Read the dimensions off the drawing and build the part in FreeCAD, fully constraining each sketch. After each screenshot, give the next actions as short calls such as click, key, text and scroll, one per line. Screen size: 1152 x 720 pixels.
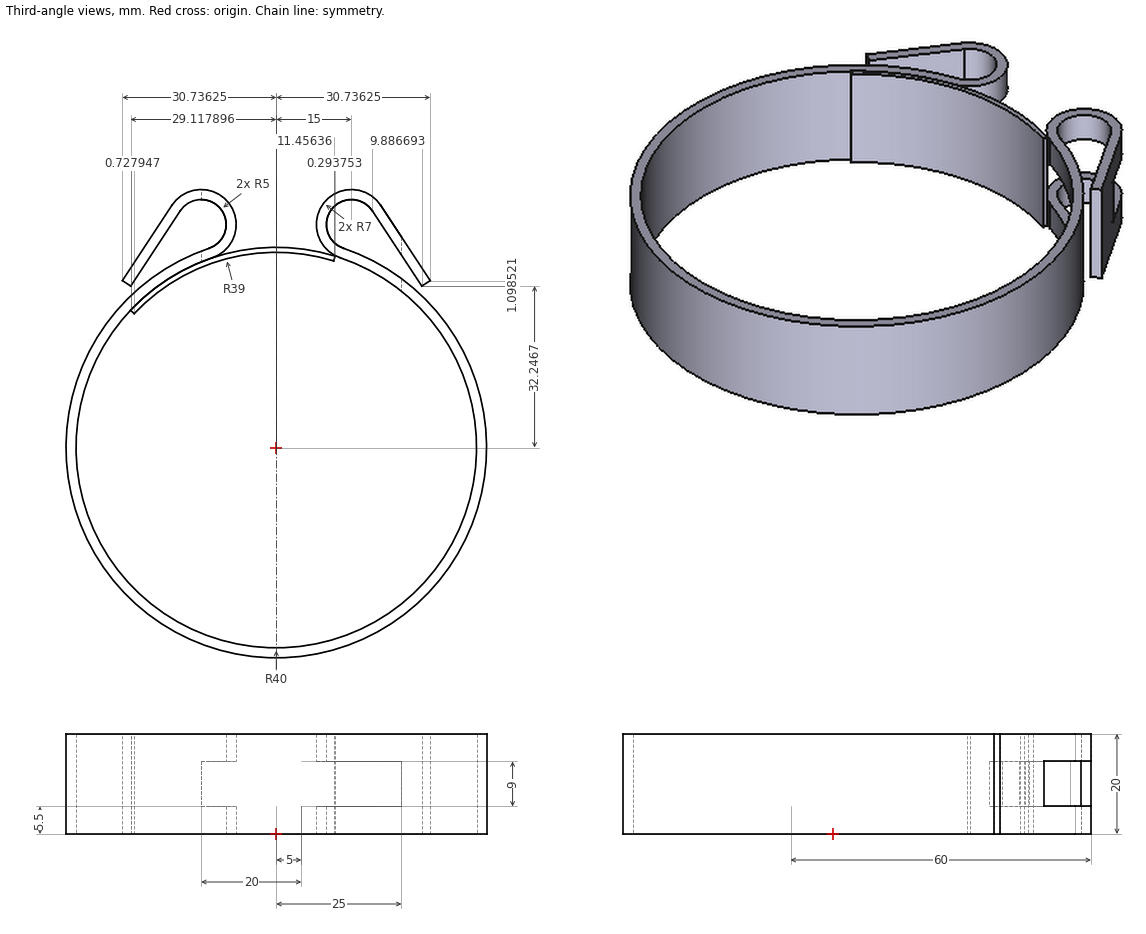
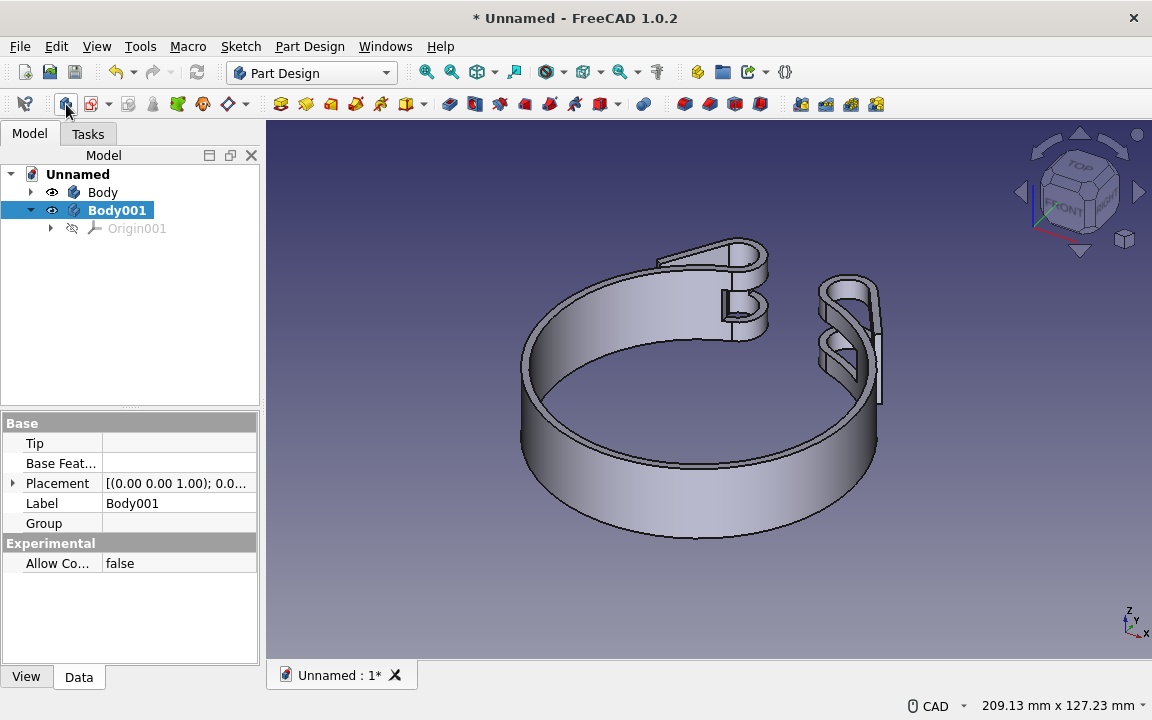
click(306, 619)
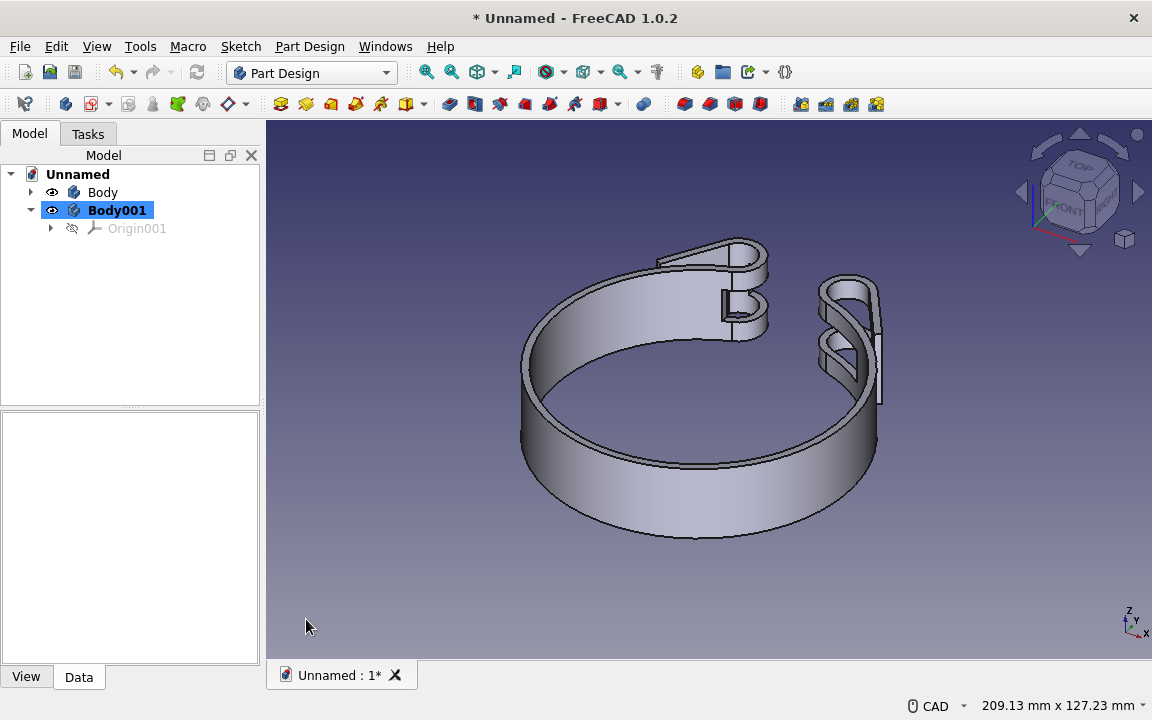
click(90, 104)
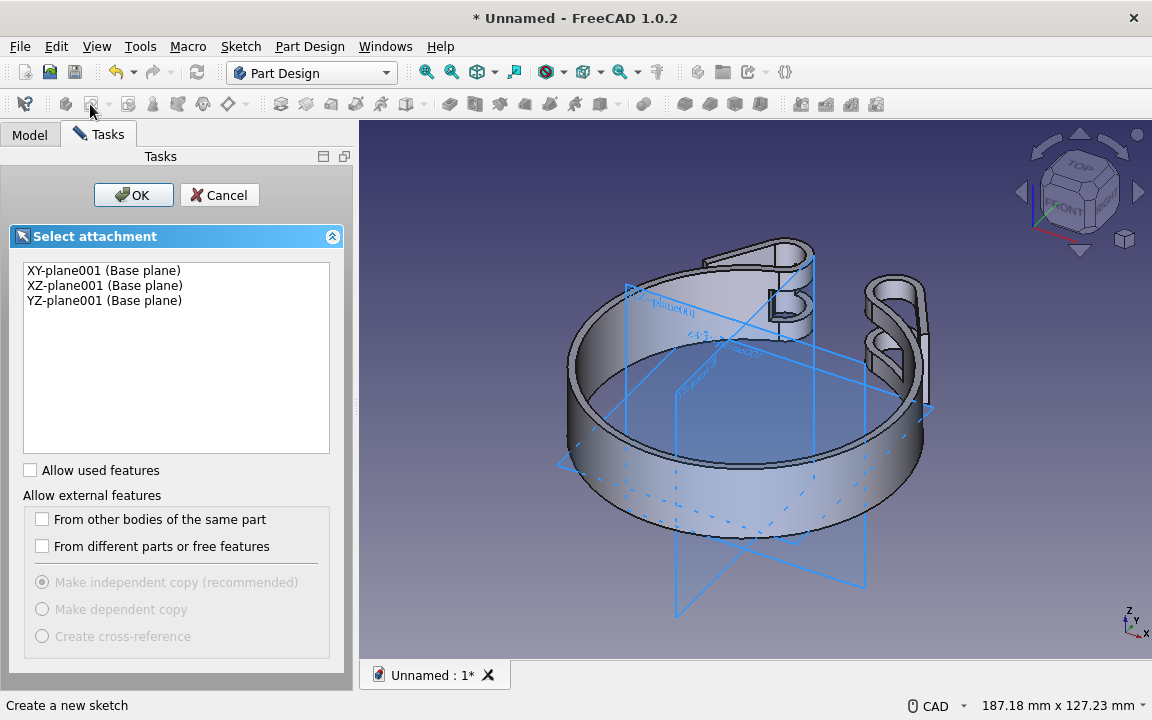
click(84, 270)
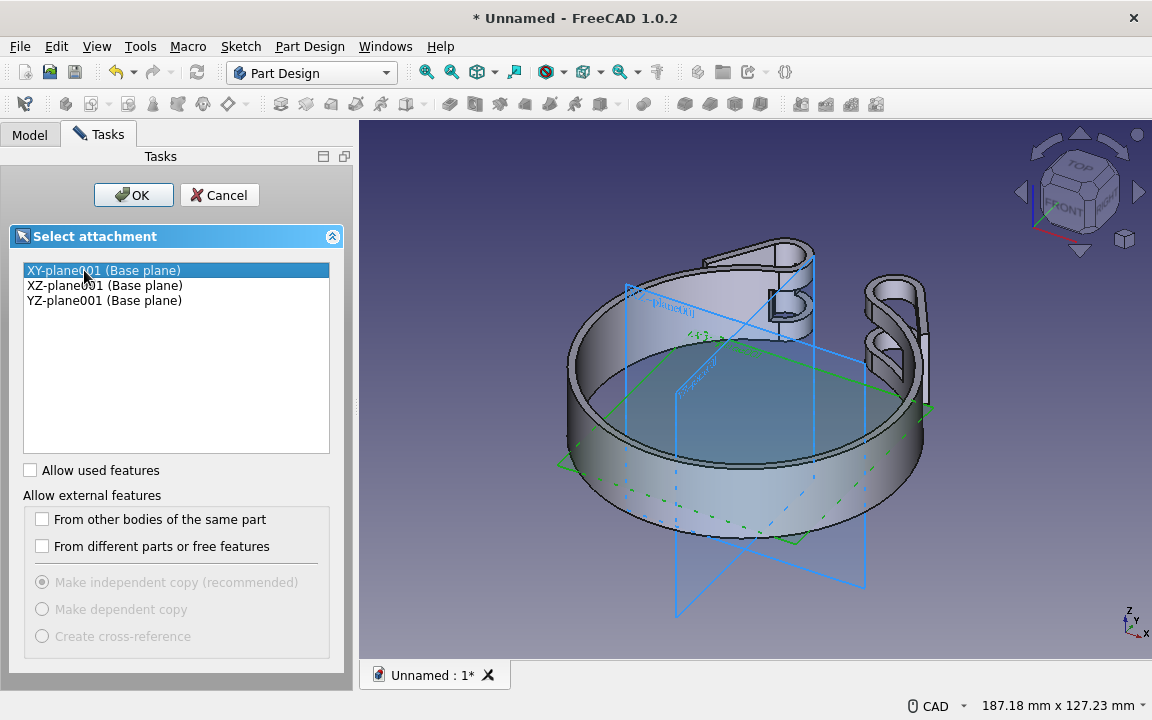
click(134, 195)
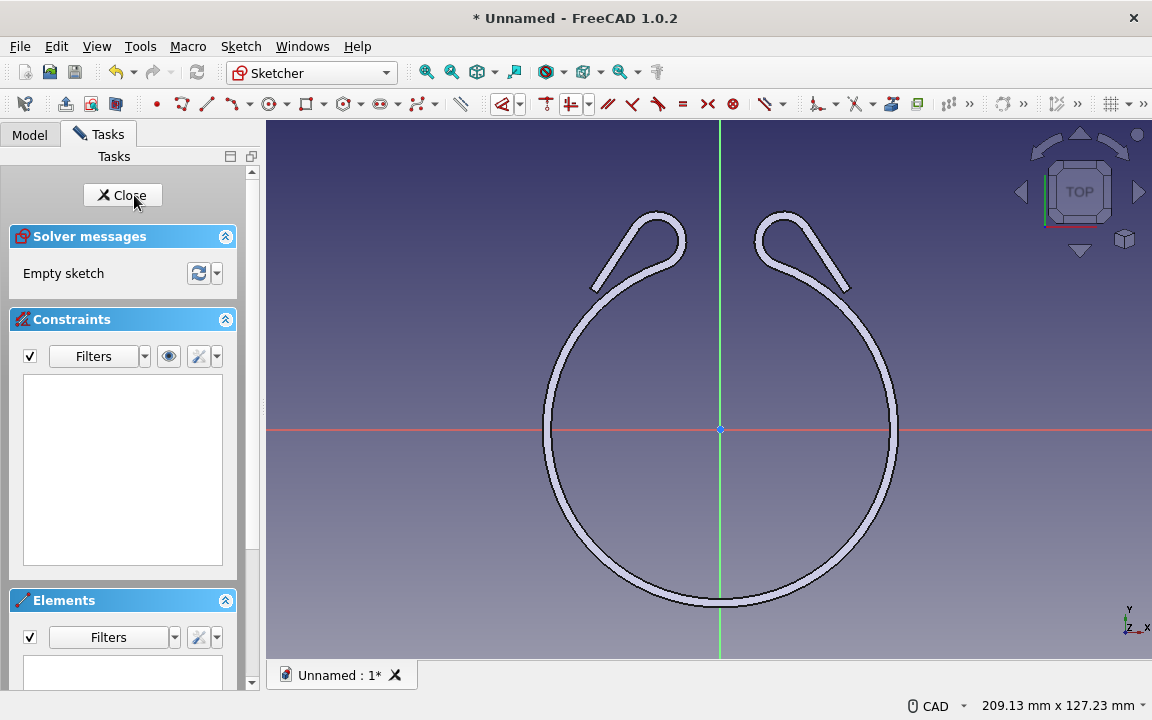
scroll(719, 314, up, 4)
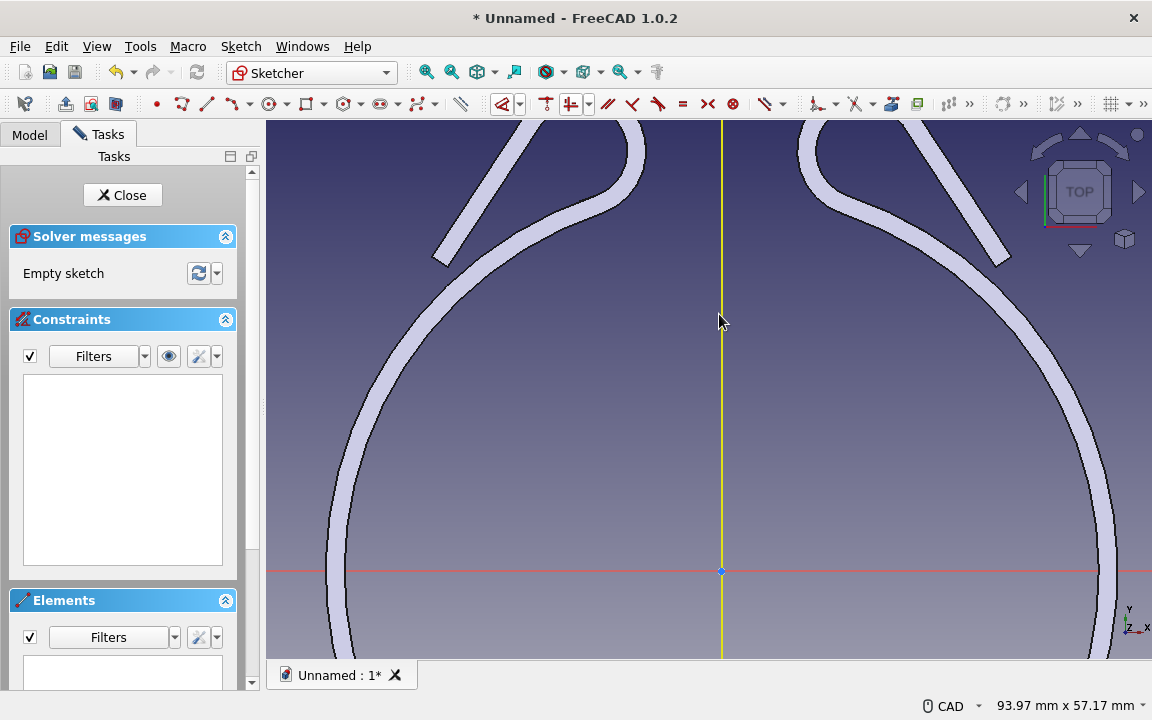
key(g)
key(l)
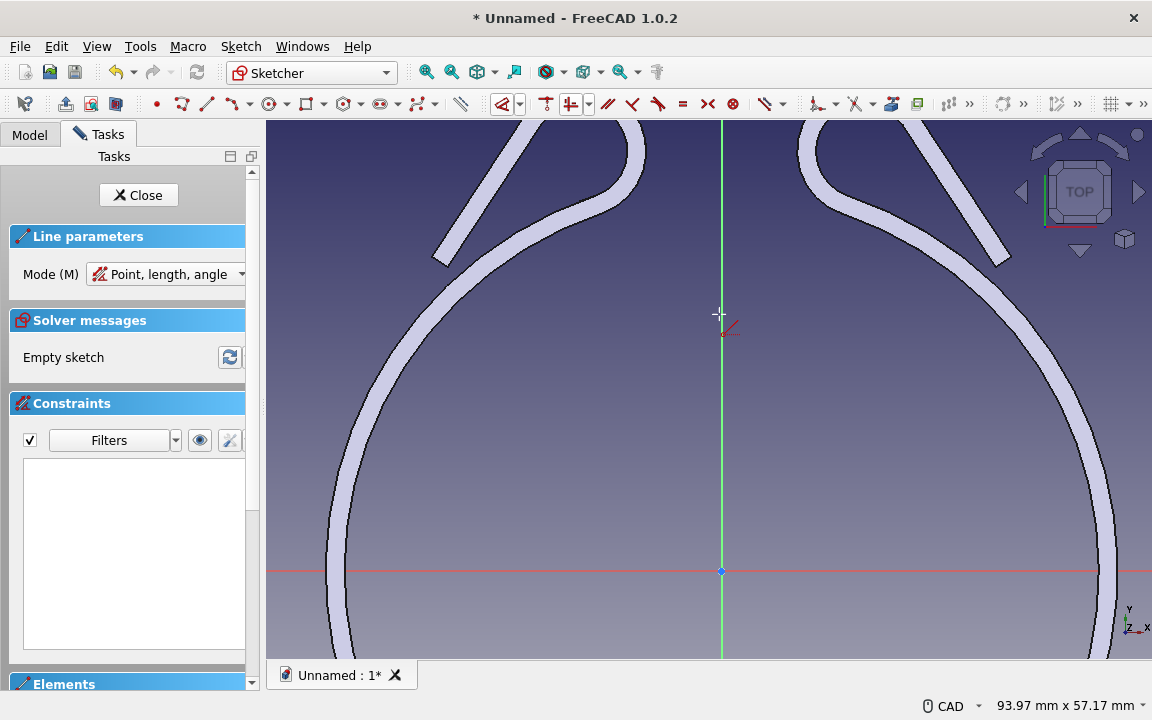
click(447, 313)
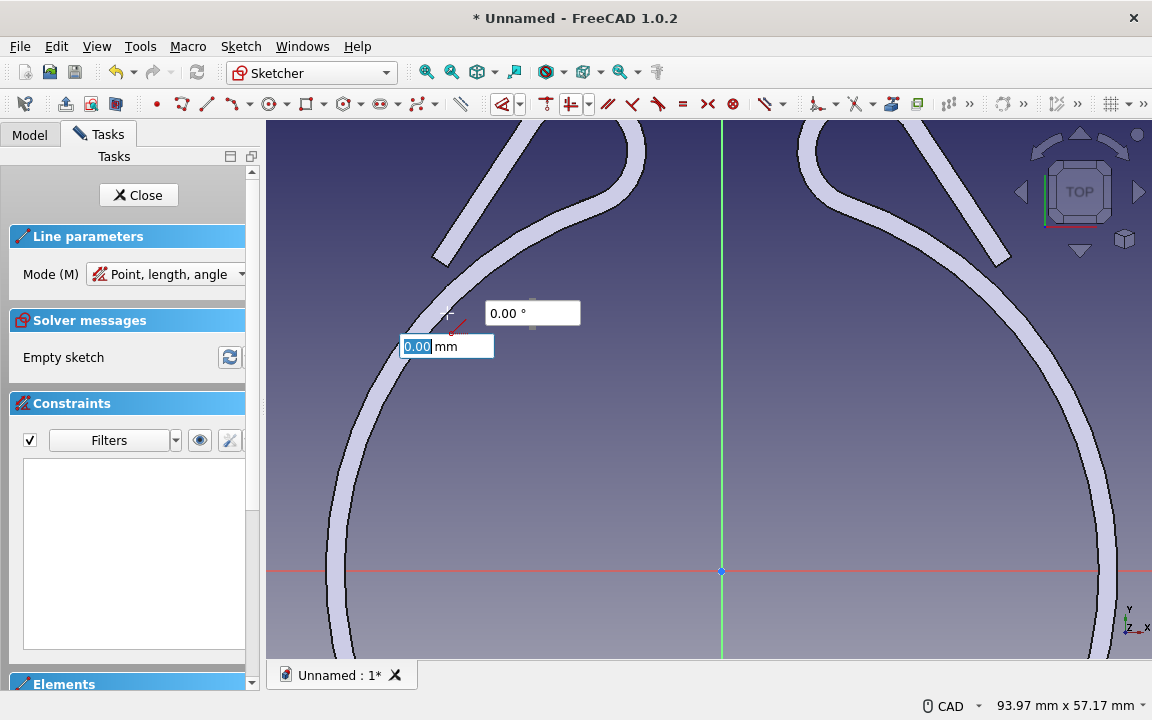
scroll(454, 319, up, 3)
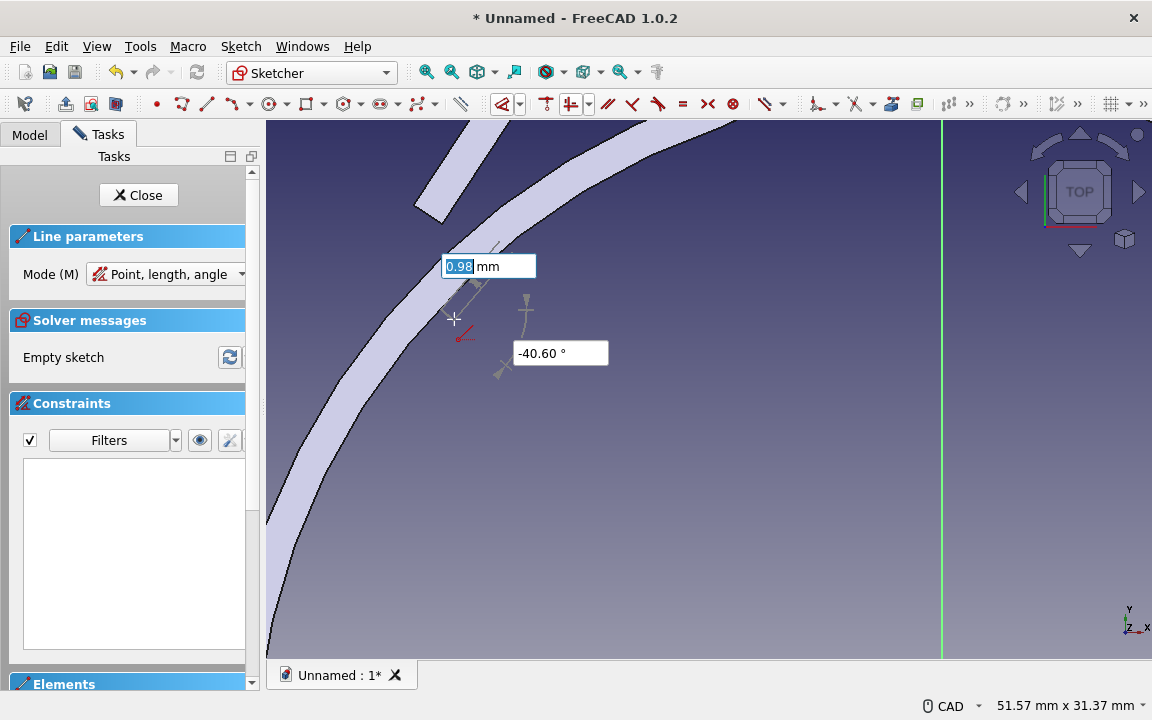
click(454, 319)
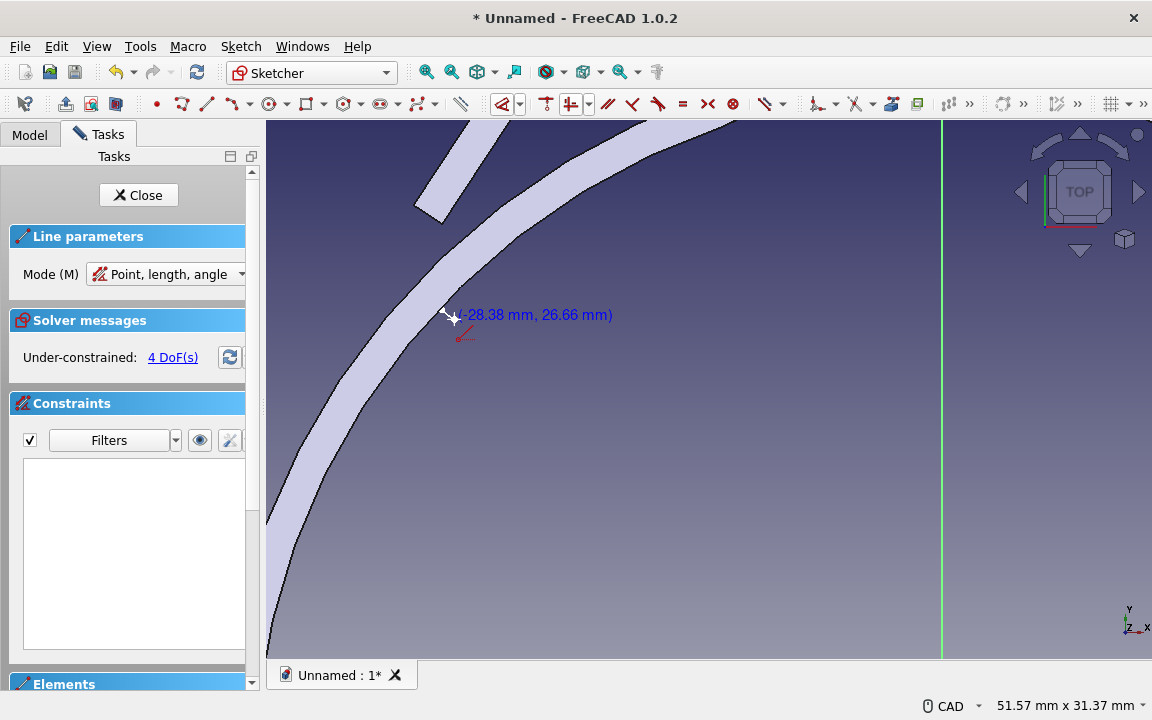
scroll(456, 321, down, 3)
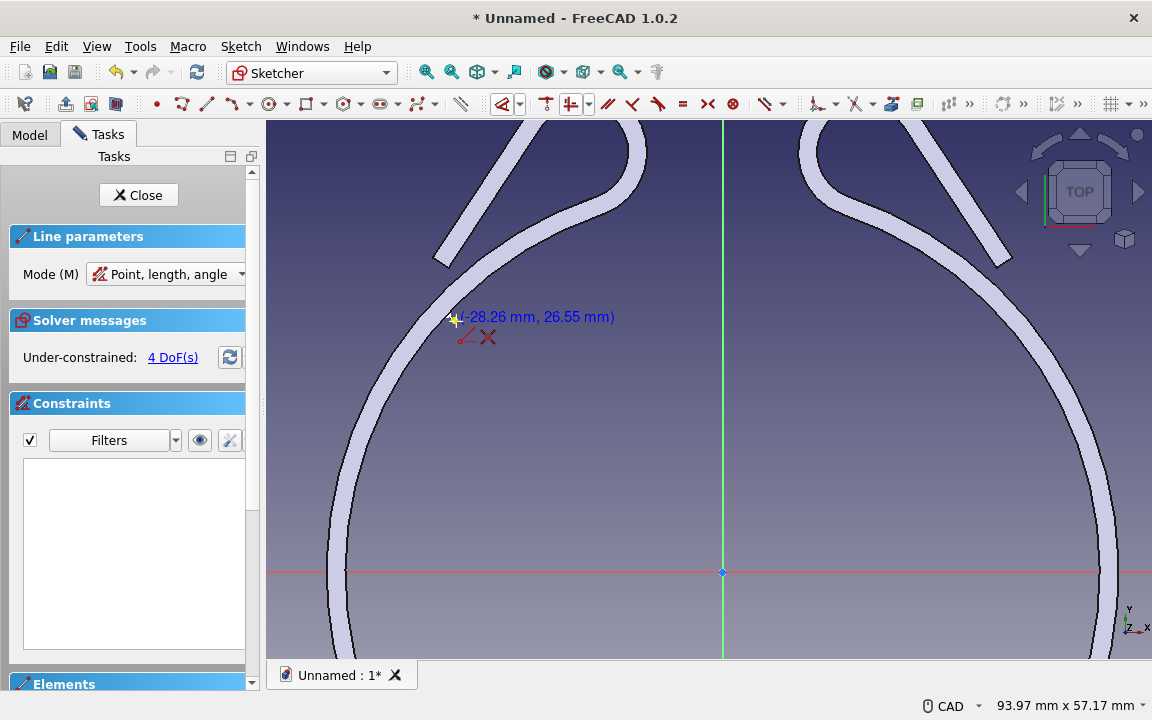
click(831, 221)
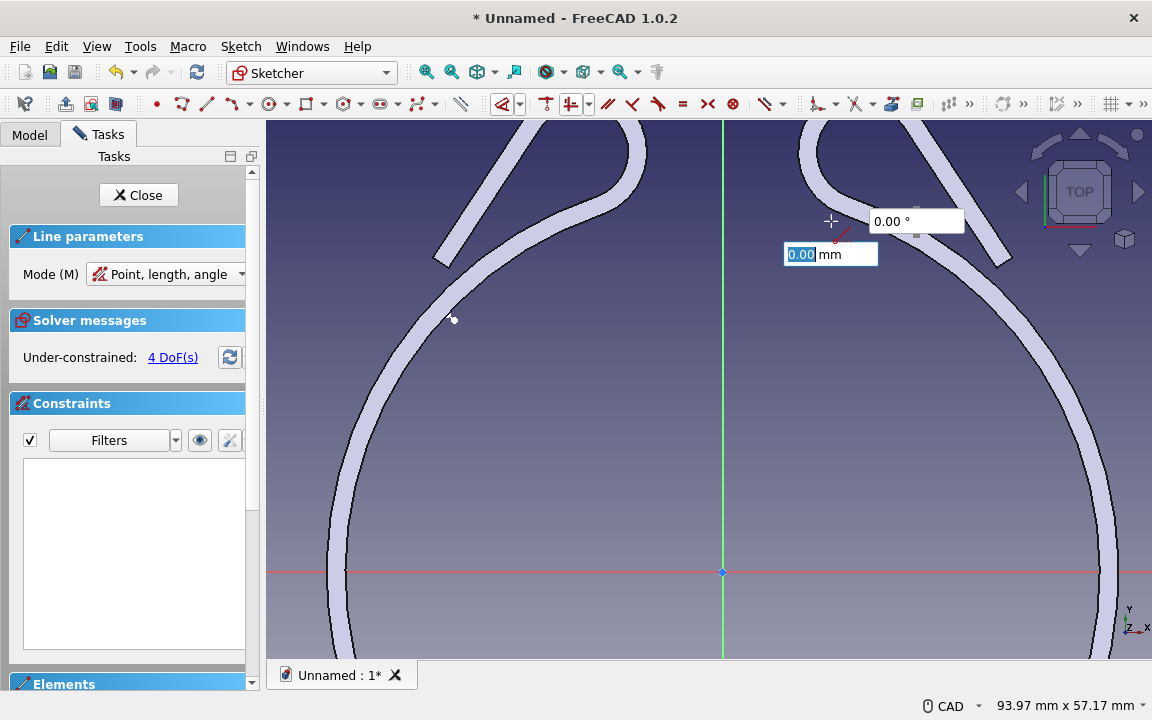
scroll(833, 212, up, 3)